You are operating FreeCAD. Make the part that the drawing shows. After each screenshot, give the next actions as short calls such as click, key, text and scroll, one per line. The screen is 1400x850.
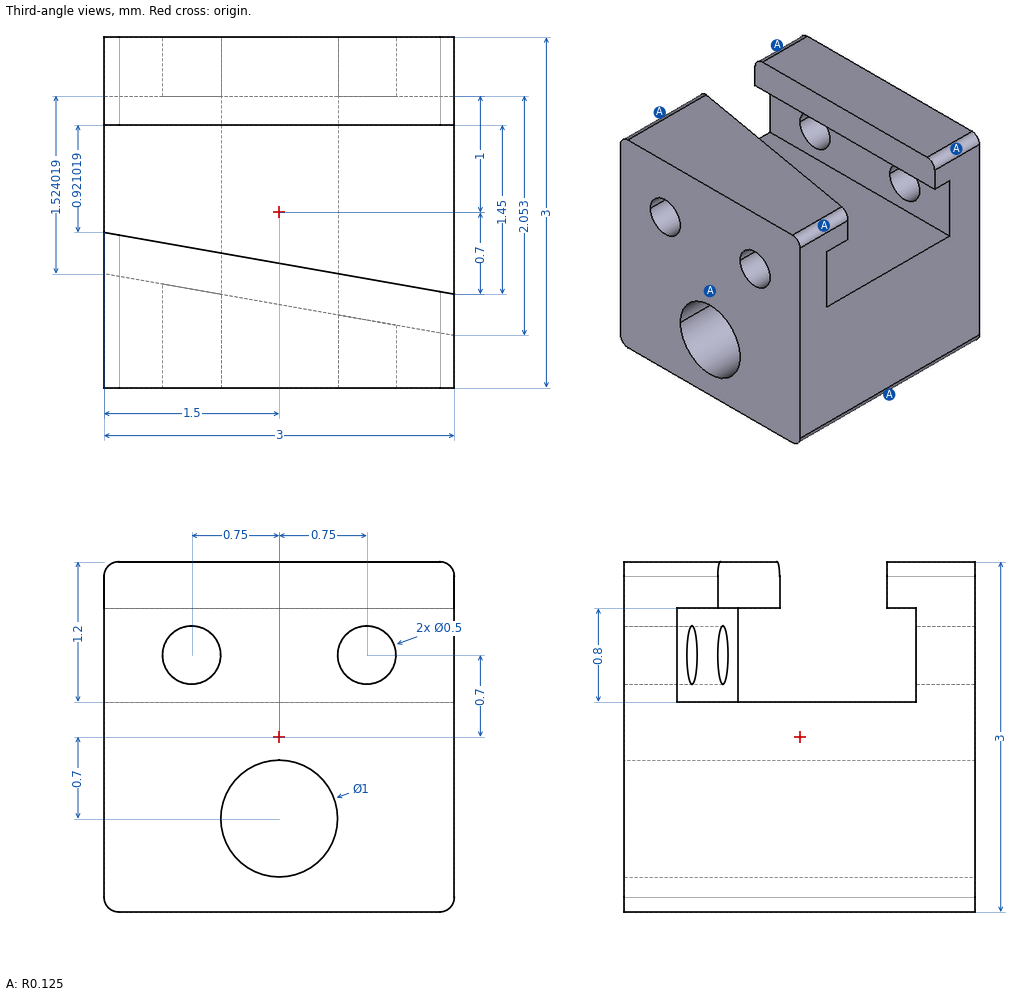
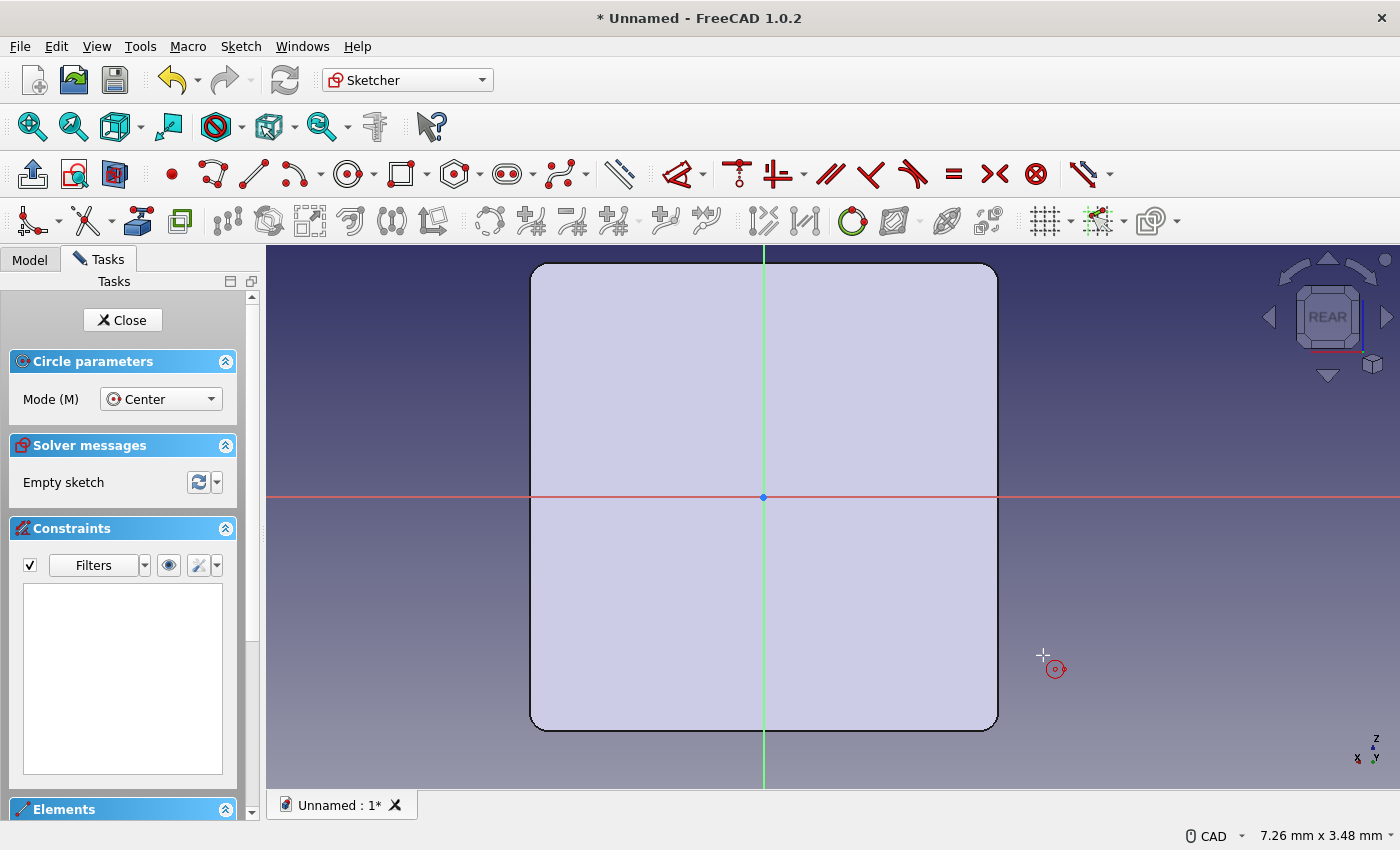
click(764, 606)
click(819, 551)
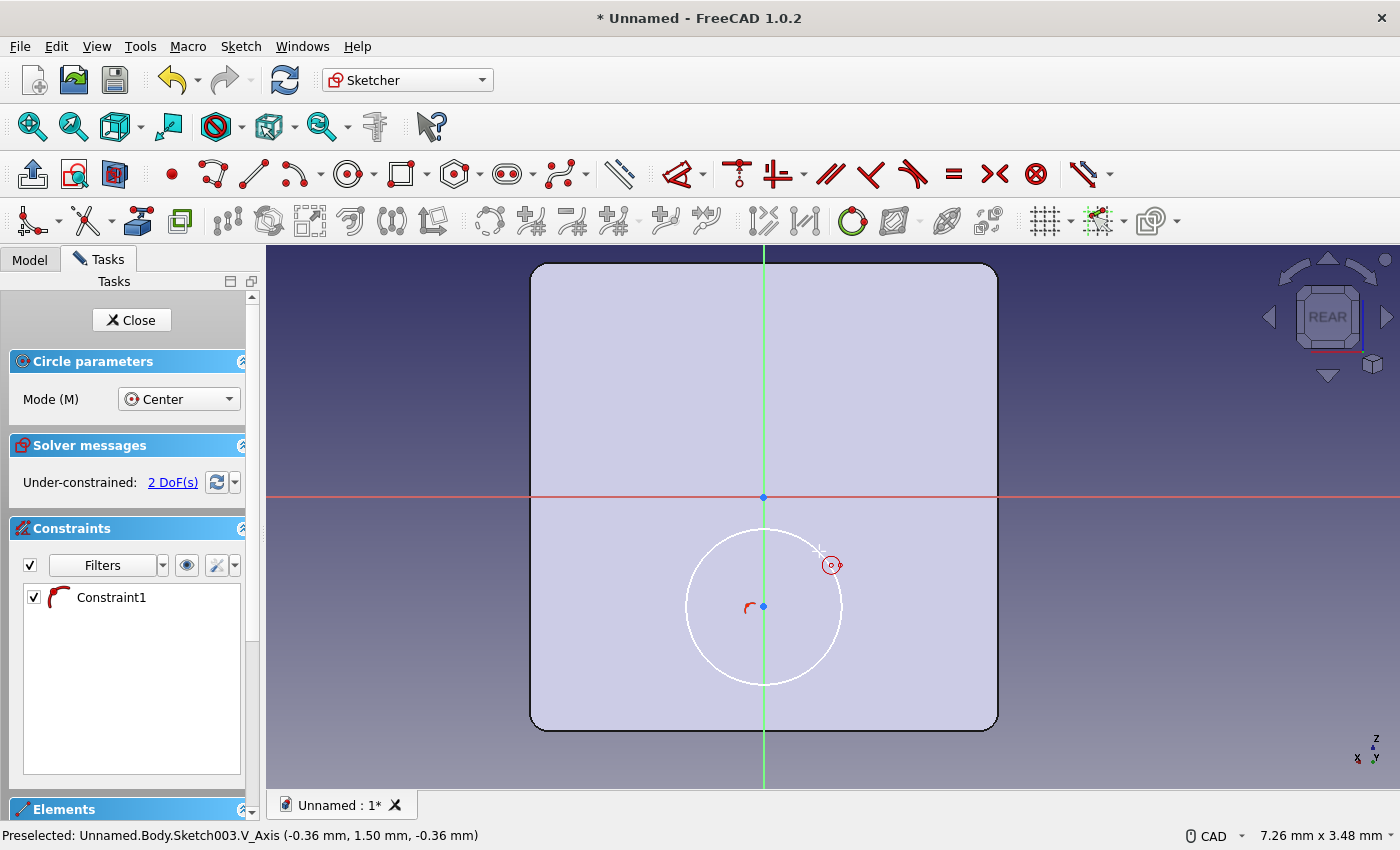
click(647, 388)
click(674, 360)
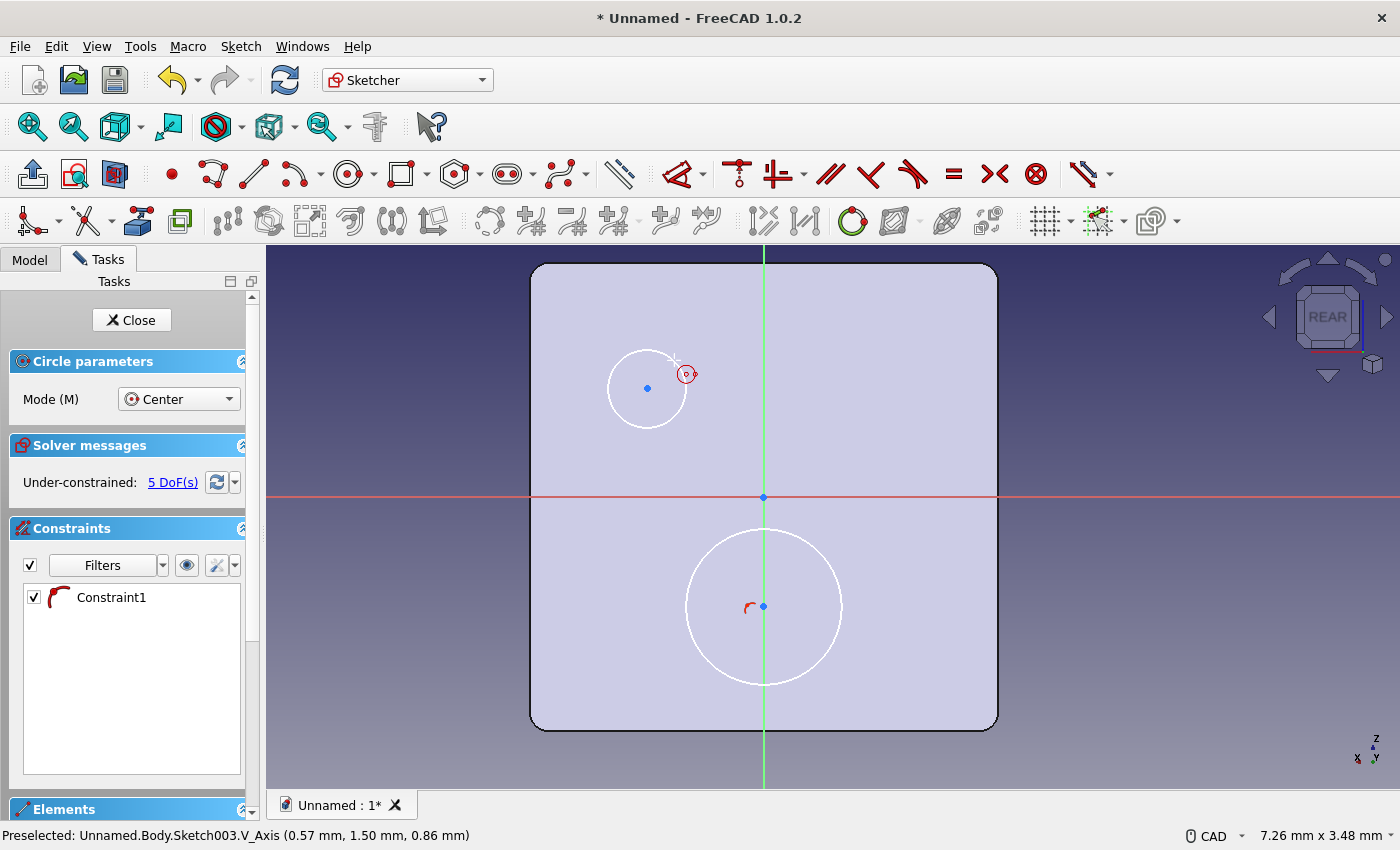
click(881, 388)
click(909, 360)
key(Escape)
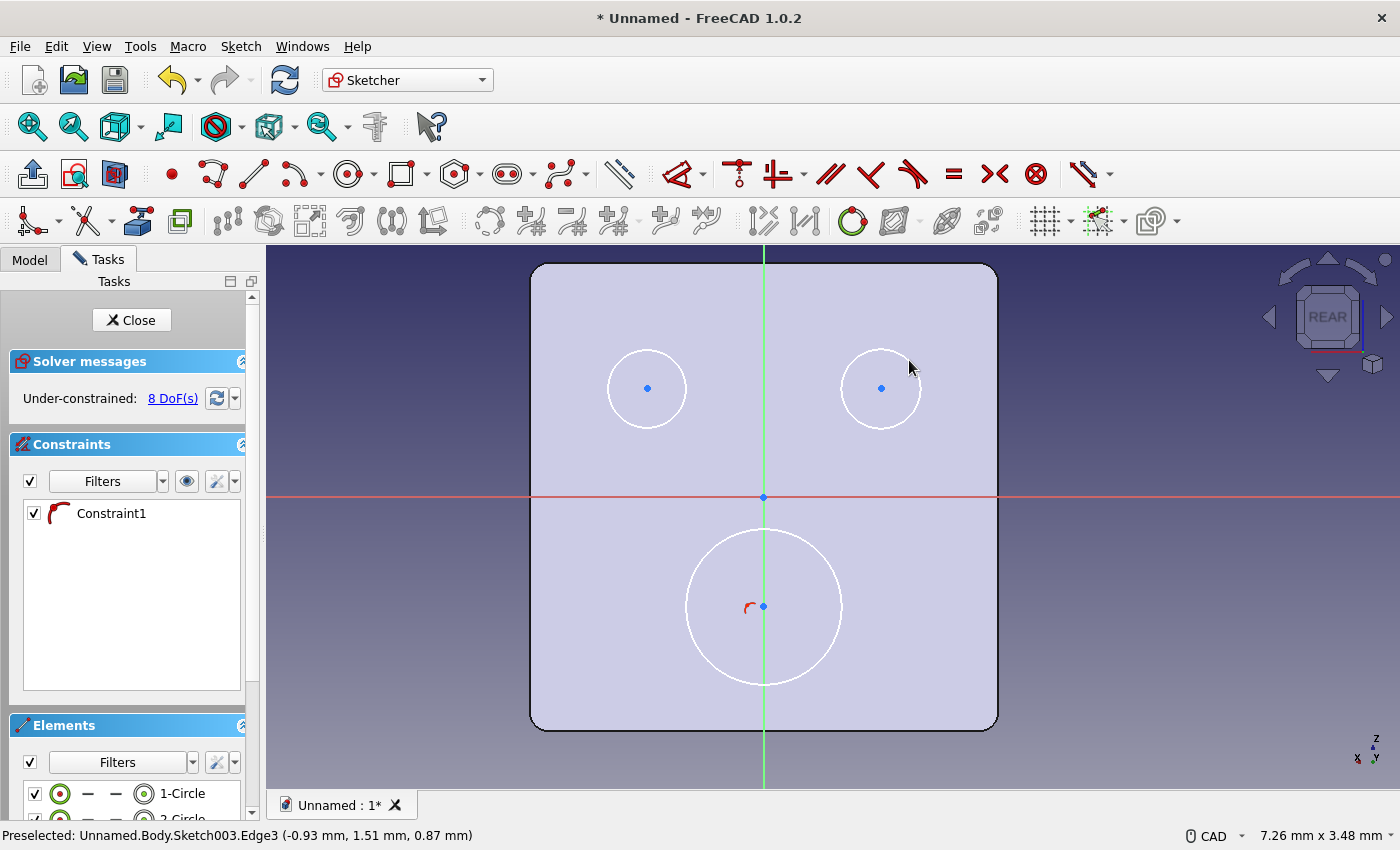
click(674, 361)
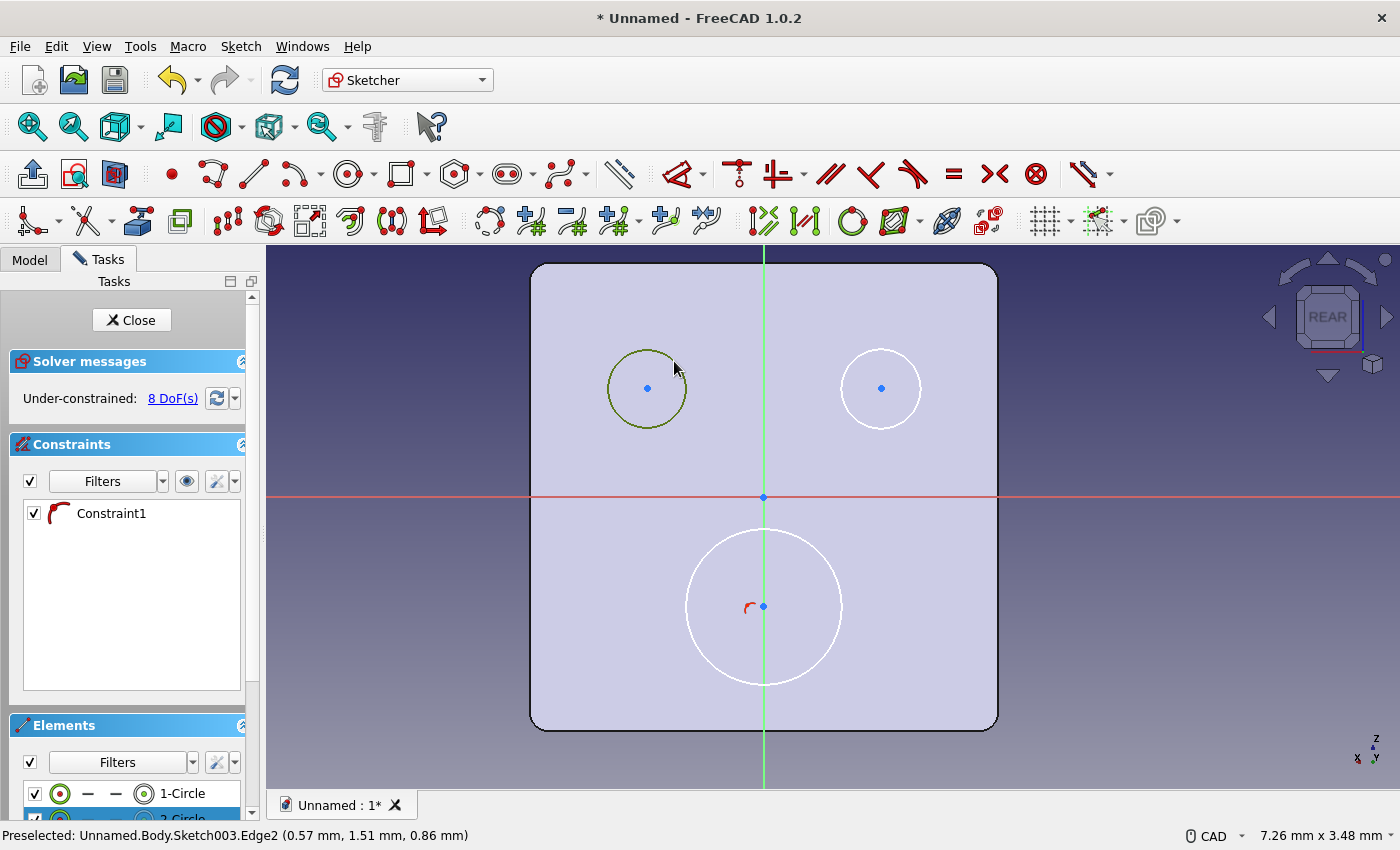
click(909, 361)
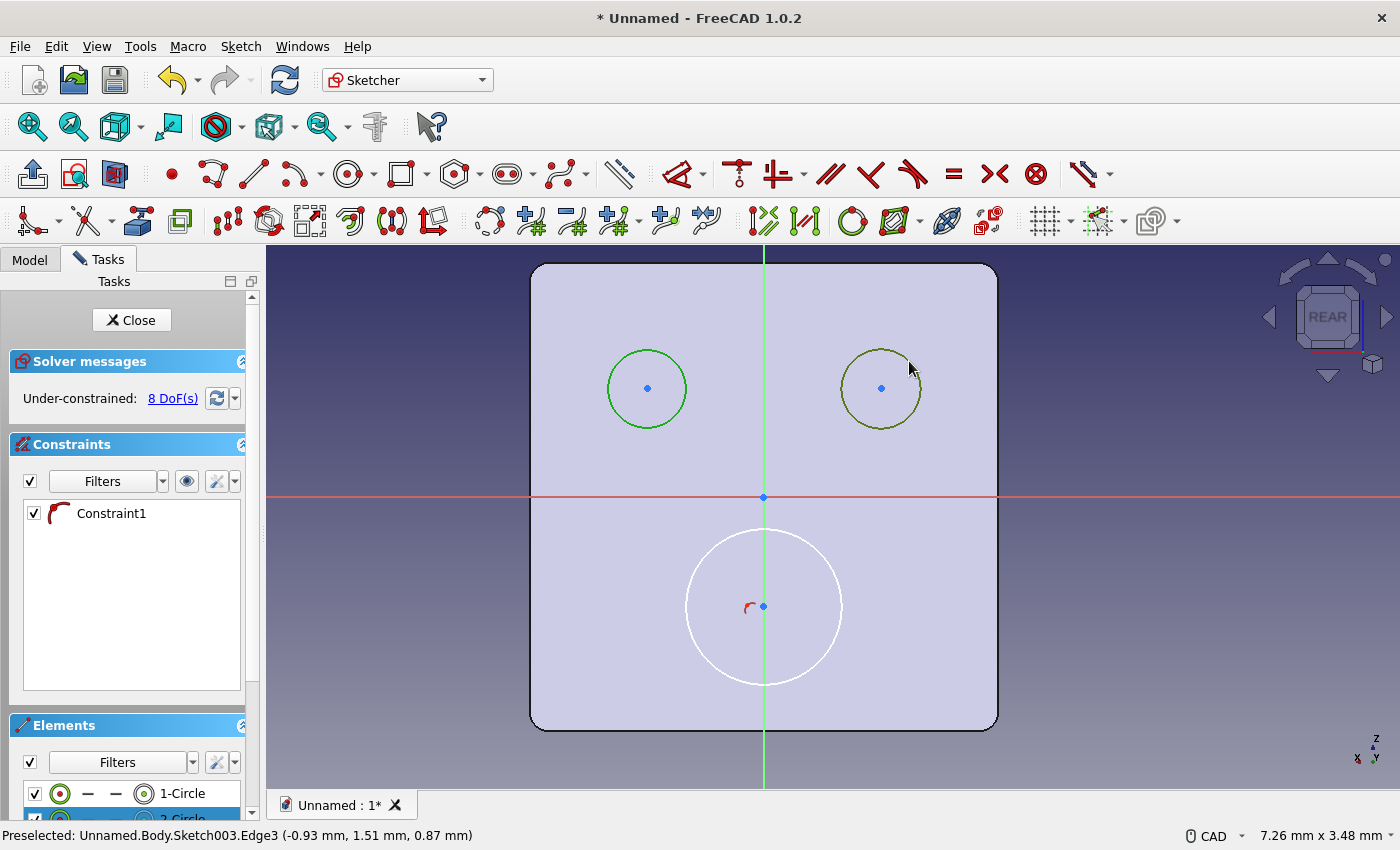
key(e)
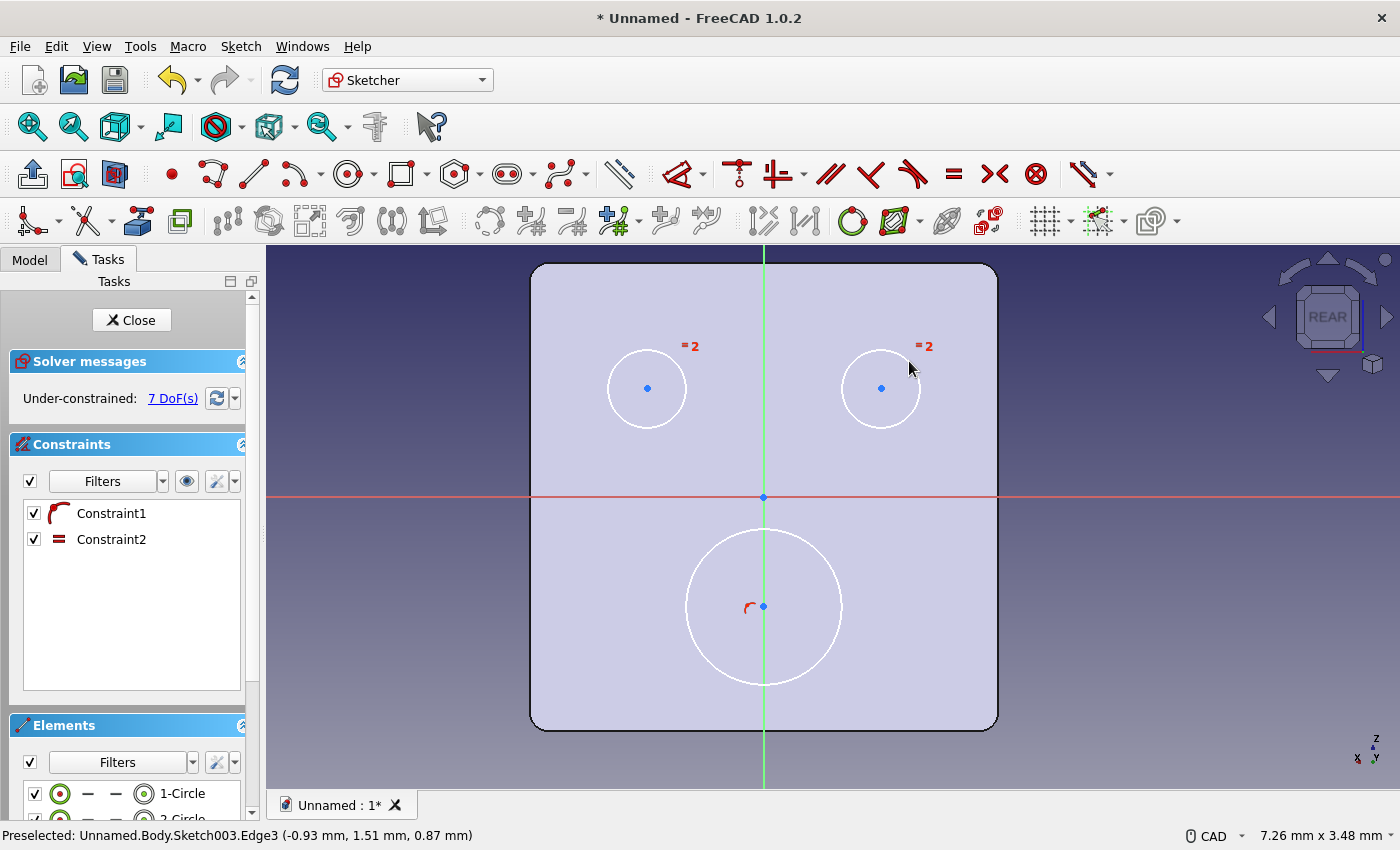
click(647, 389)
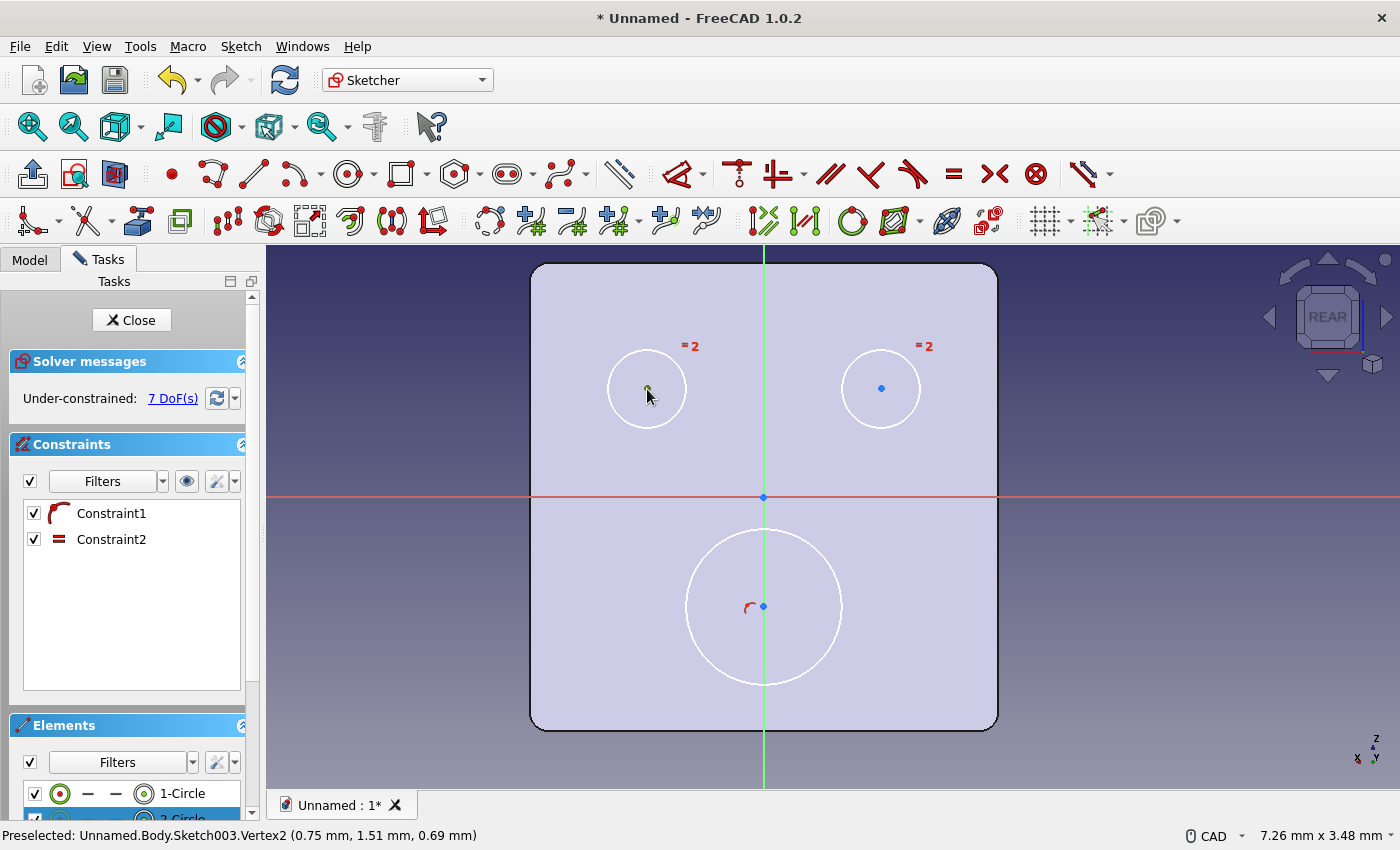
click(881, 389)